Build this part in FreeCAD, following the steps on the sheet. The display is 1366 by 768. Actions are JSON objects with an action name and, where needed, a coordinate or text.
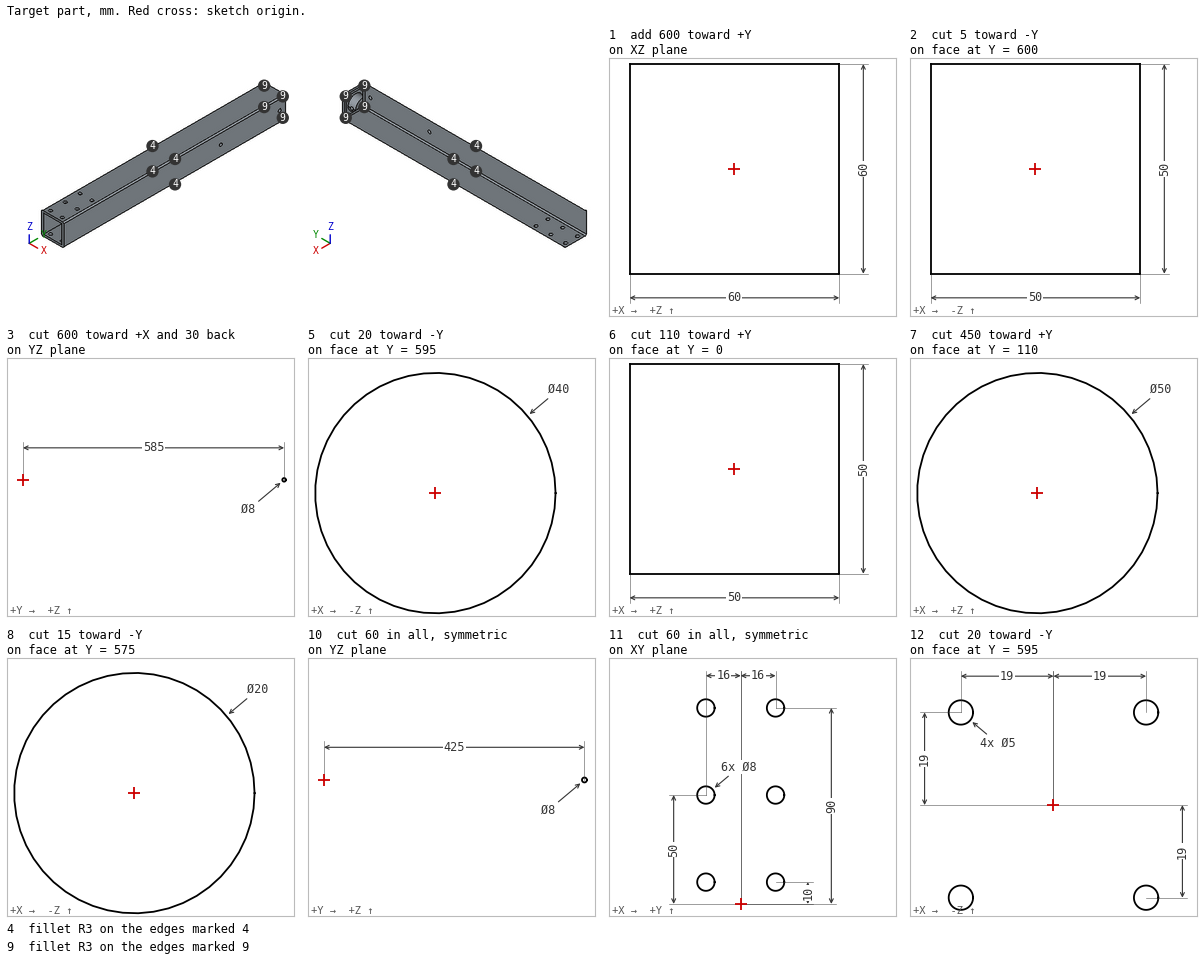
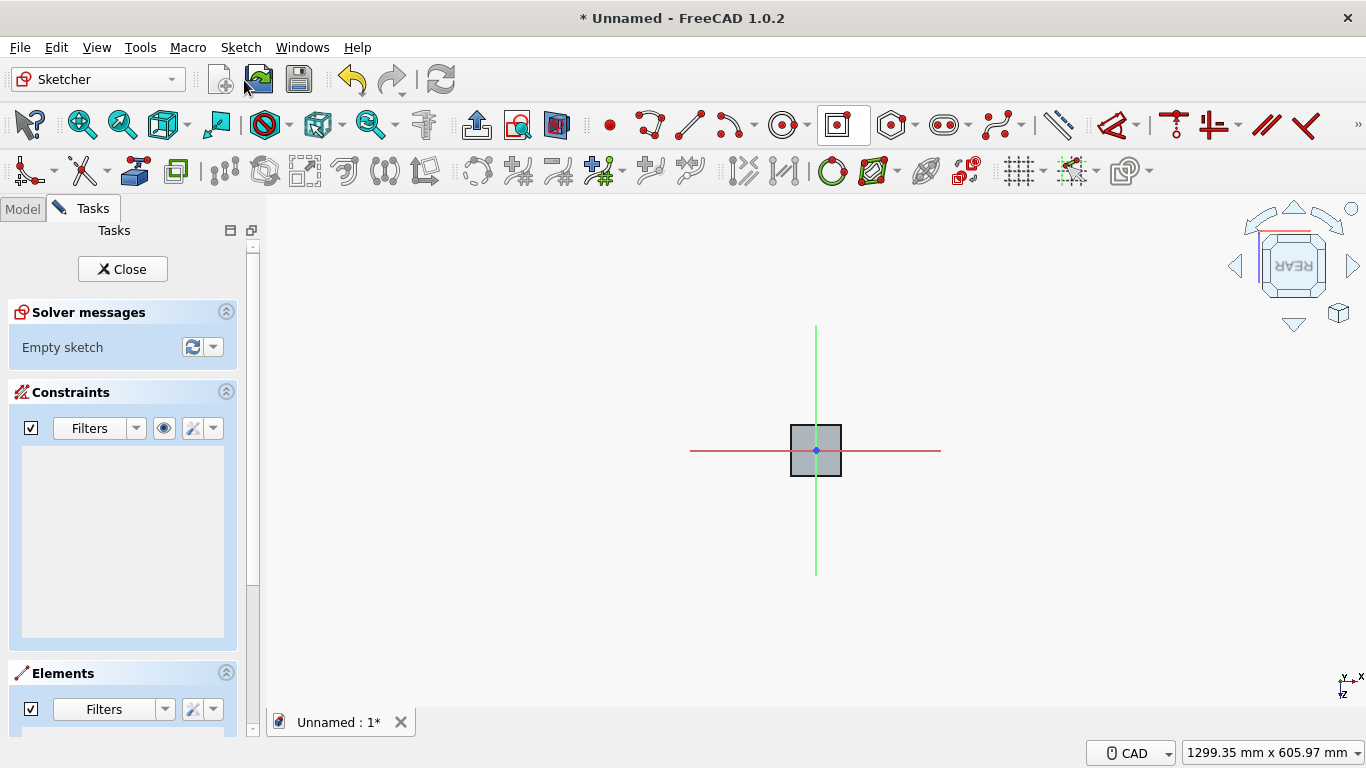
{"action": "scroll", "coordinate": [827, 450], "scroll_direction": "up", "scroll_amount": 10}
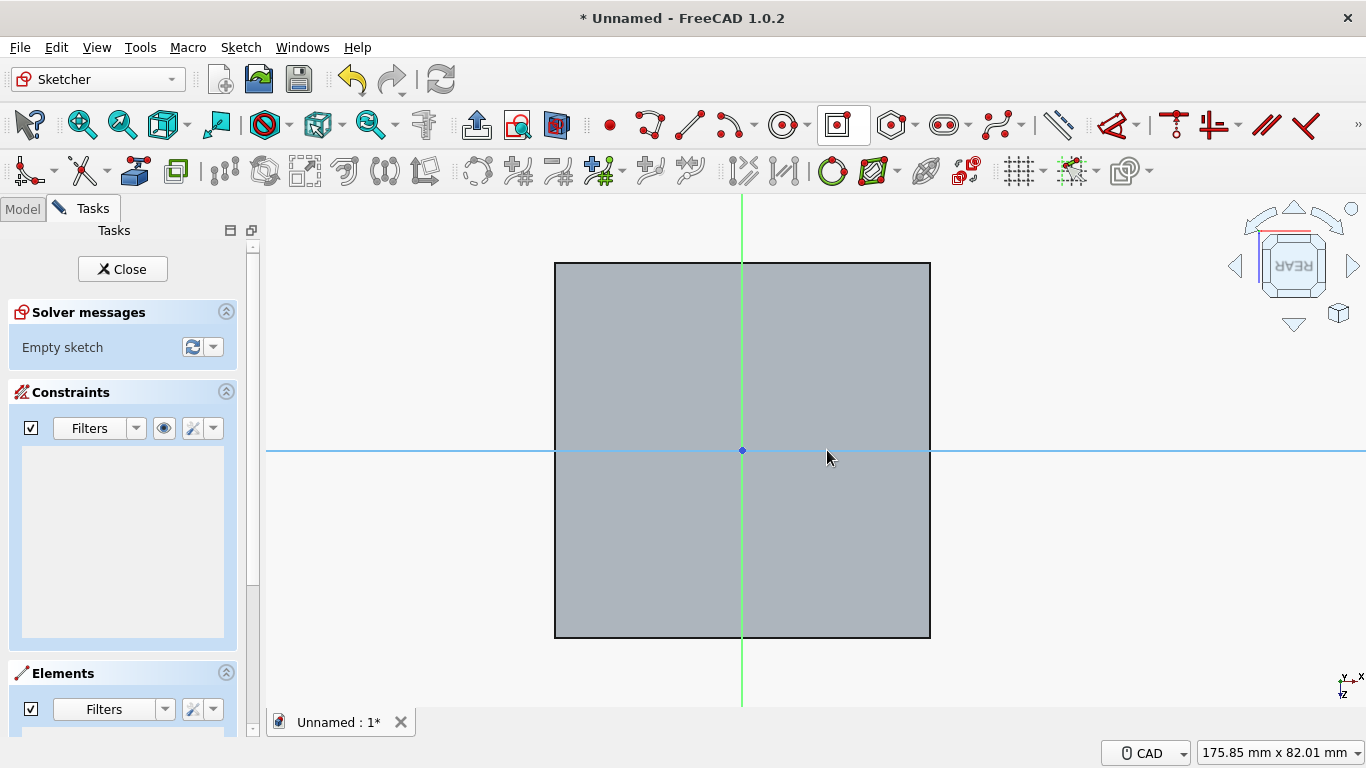
{"action": "left_click", "coordinate": [838, 126]}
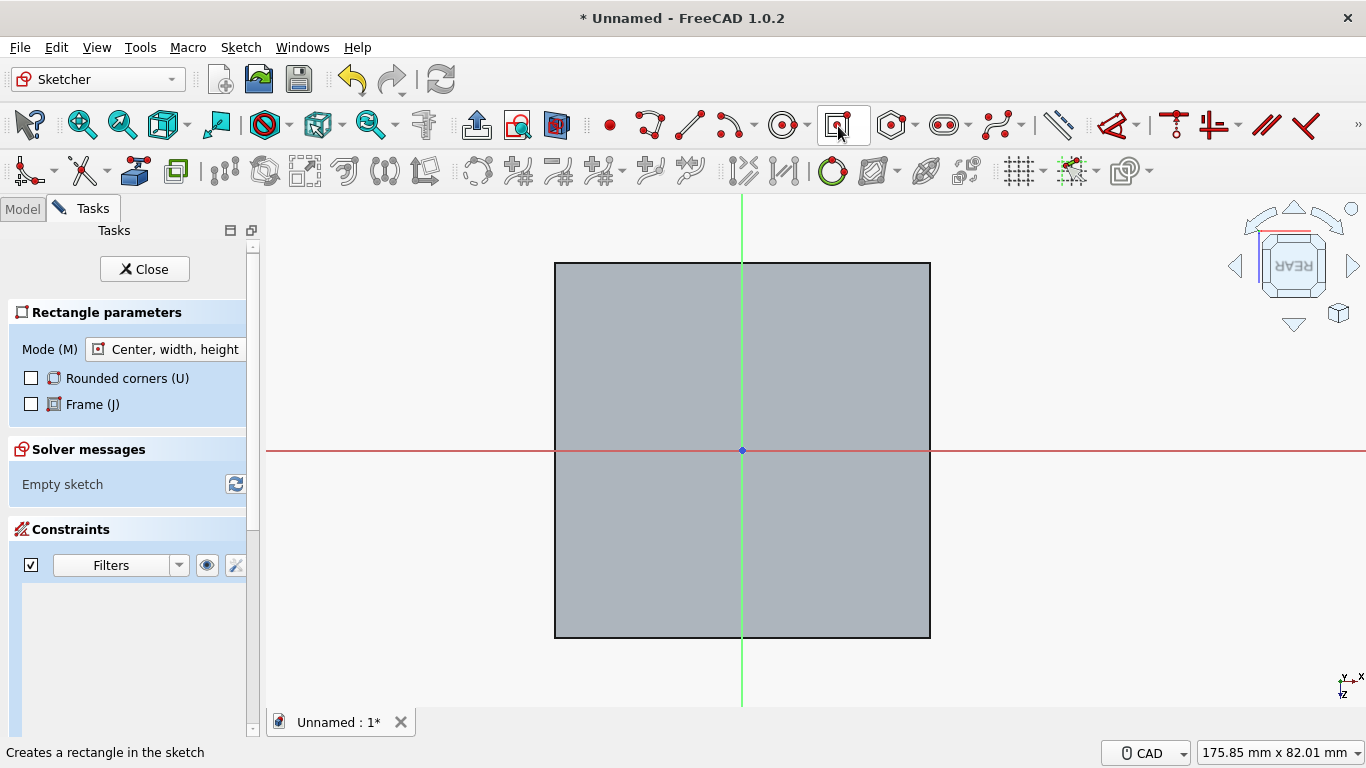
{"action": "left_click", "coordinate": [742, 450]}
{"action": "mouse_move", "coordinate": [899, 294]}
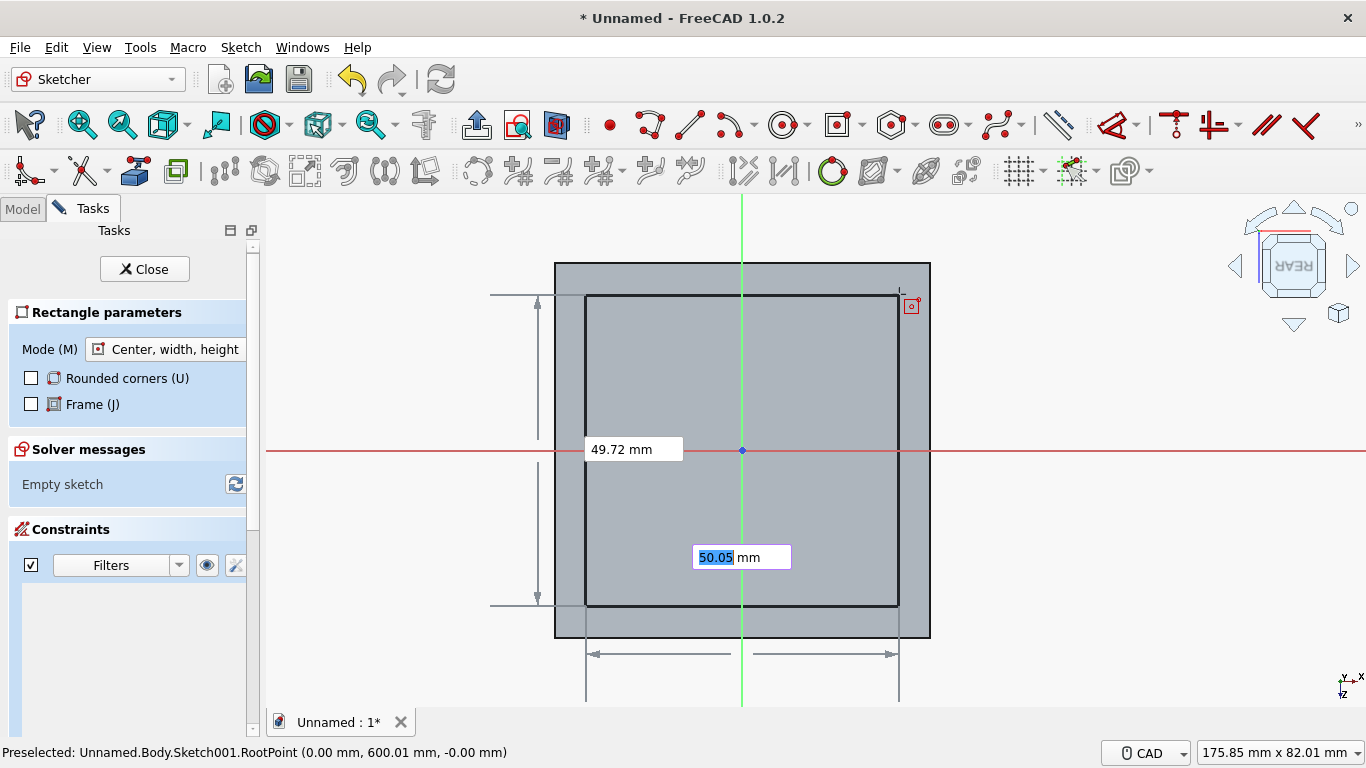
{"action": "type", "text": "50"}
{"action": "key", "text": "Tab"}
{"action": "type", "text": "50"}
{"action": "key", "text": "Return"}
{"action": "key", "text": "Escape"}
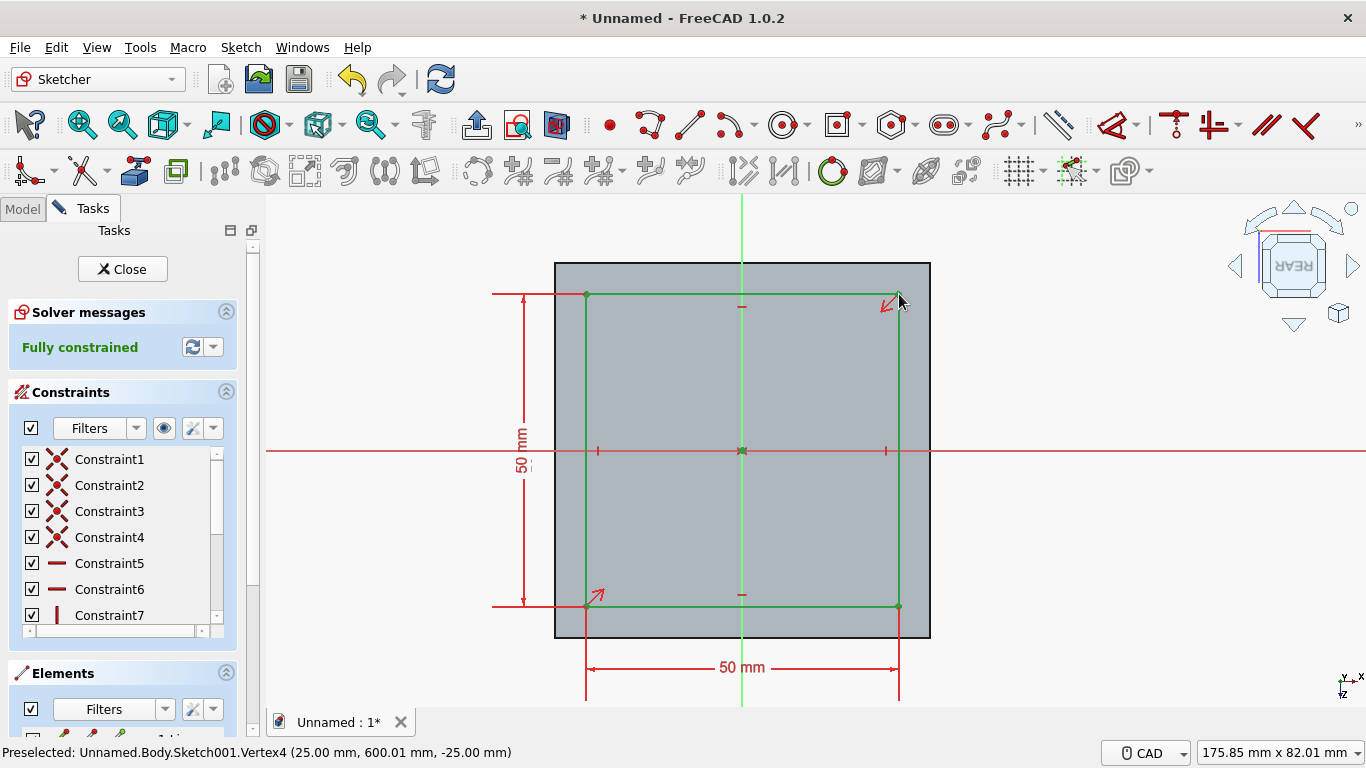
{"action": "left_click", "coordinate": [123, 269]}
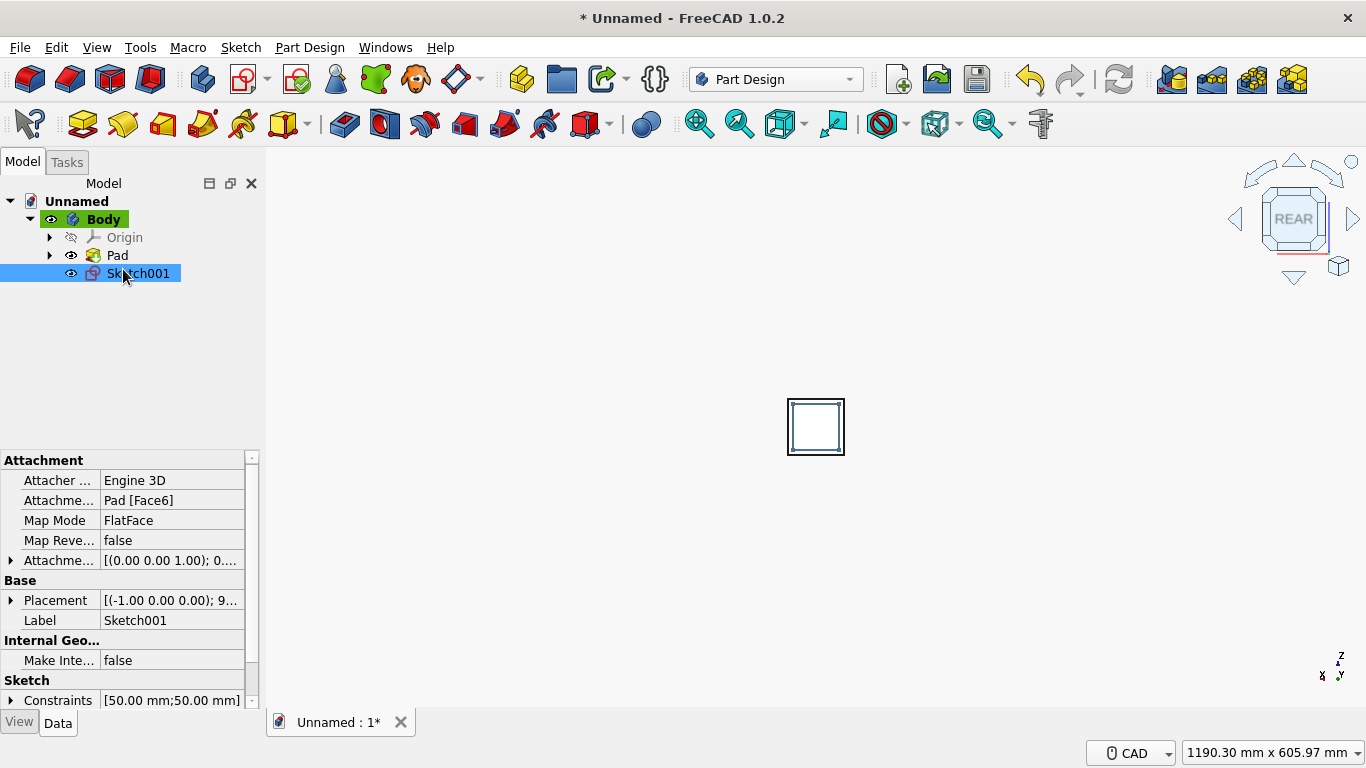
{"action": "left_click", "coordinate": [346, 124]}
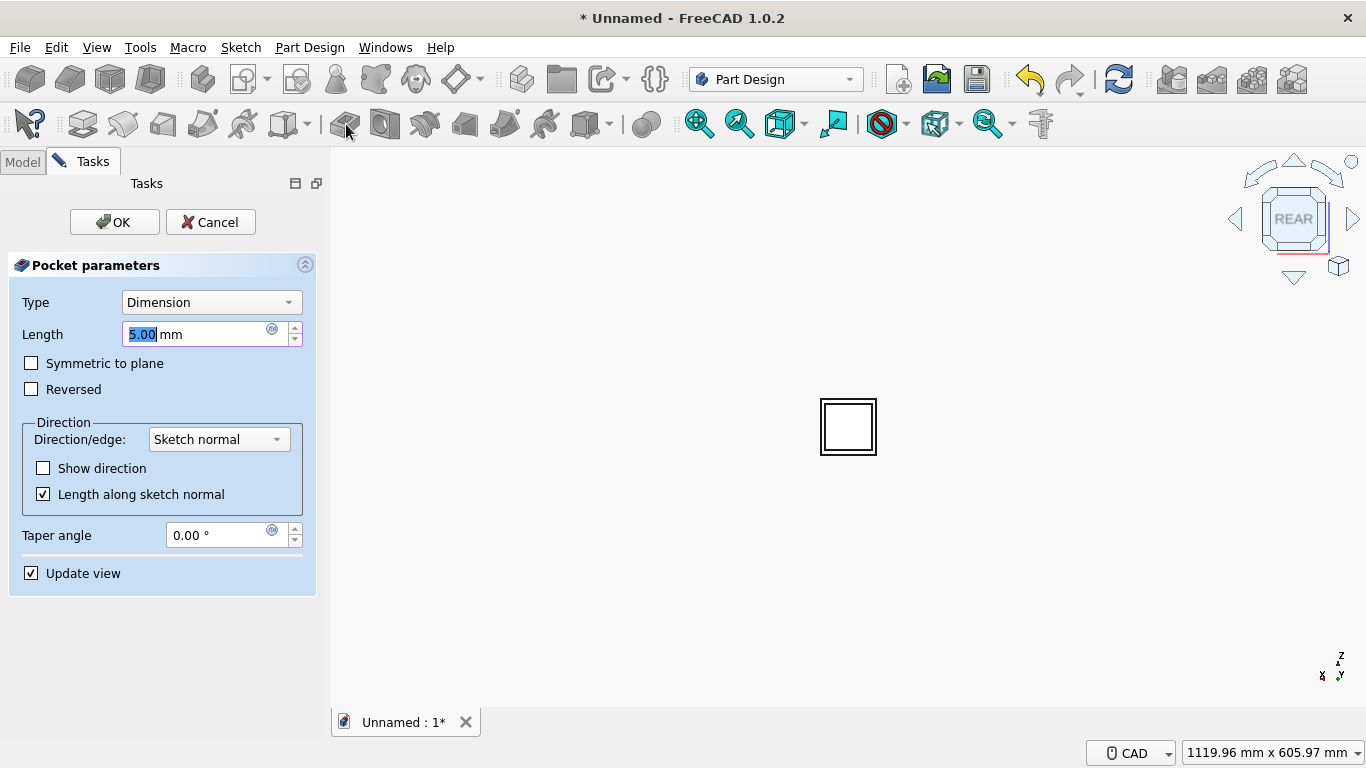
{"action": "type", "text": "5"}
{"action": "key", "text": "Tab"}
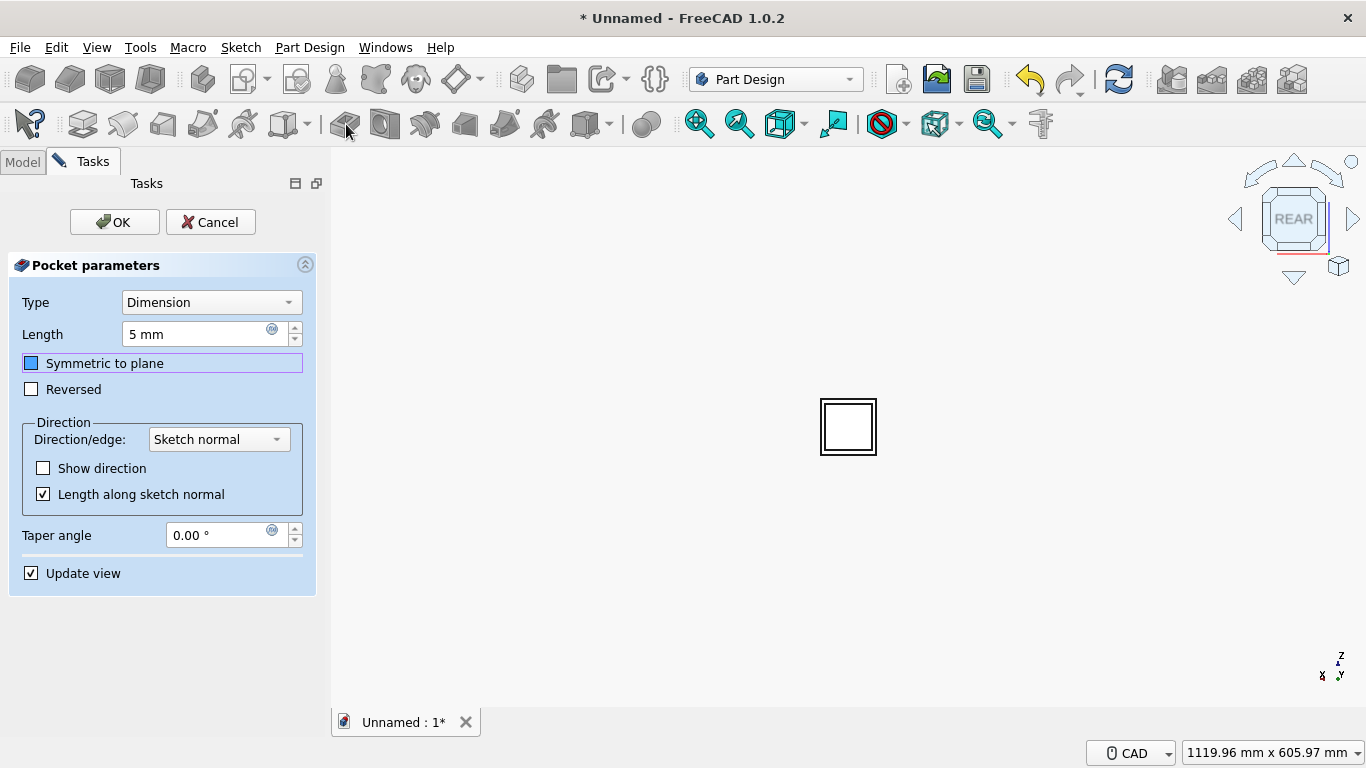
{"action": "left_click", "coordinate": [115, 222]}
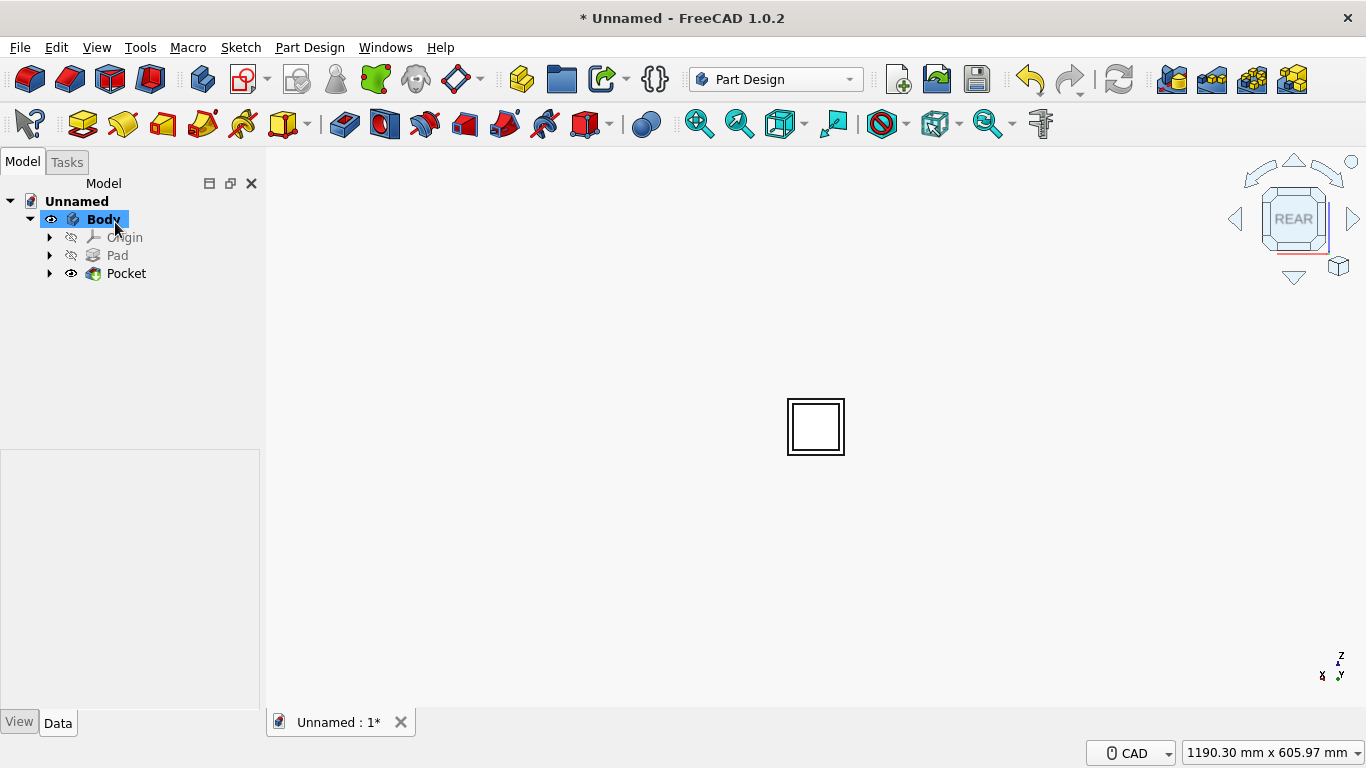
{"action": "key", "text": "v f"}